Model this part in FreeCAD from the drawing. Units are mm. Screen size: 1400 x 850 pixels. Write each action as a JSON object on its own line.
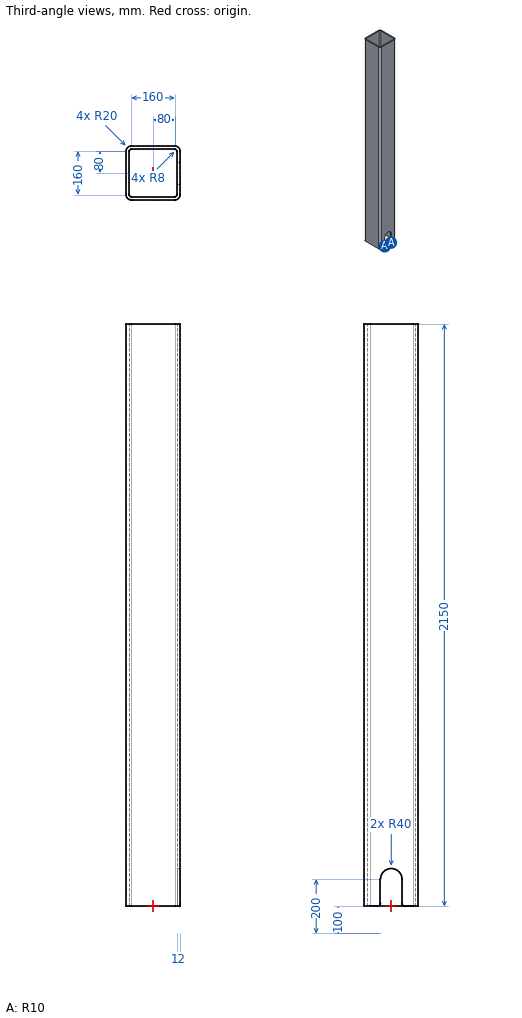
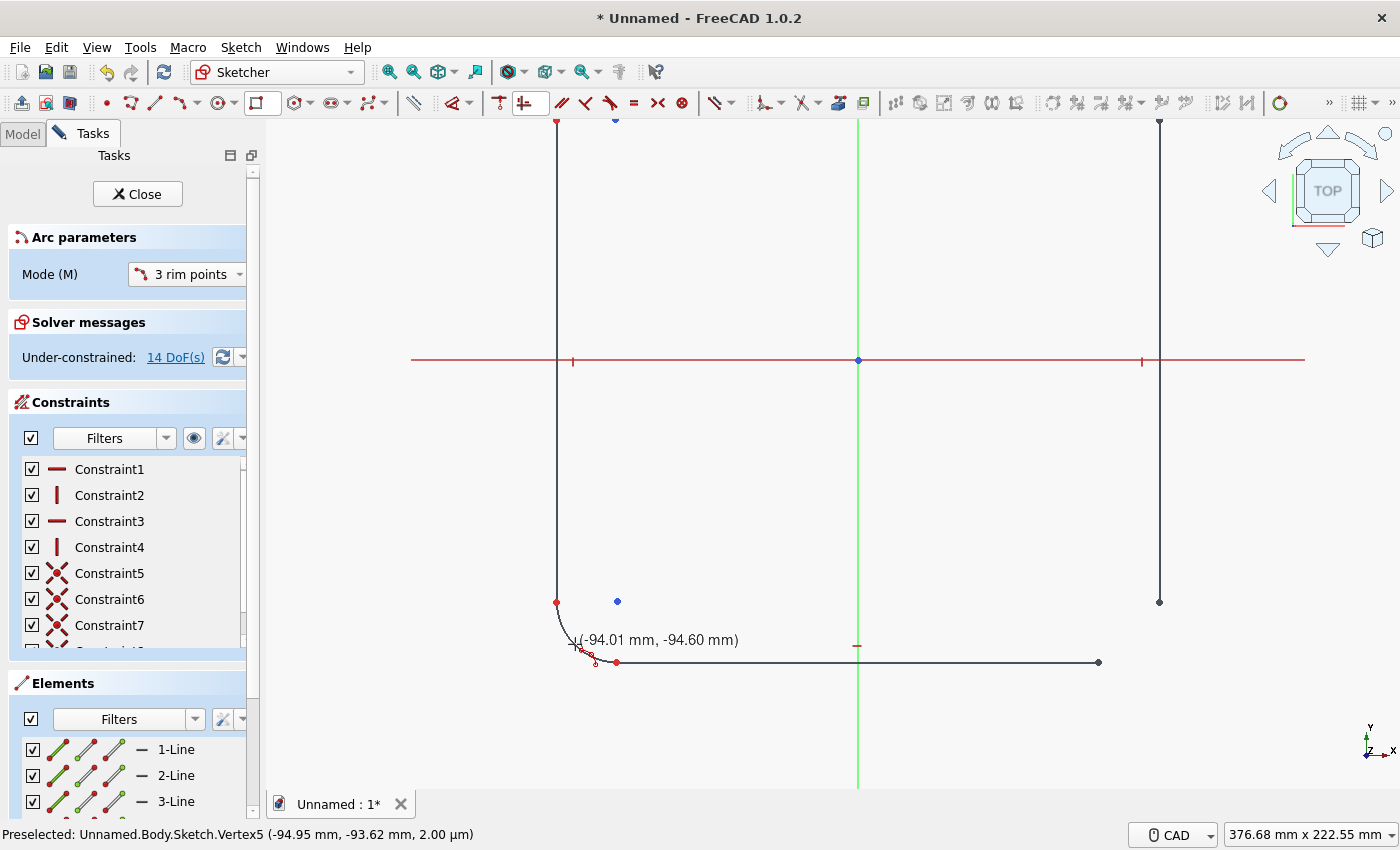
{"action": "left_click", "coordinate": [1098, 663]}
{"action": "left_click", "coordinate": [1160, 603]}
{"action": "left_click", "coordinate": [1141, 644]}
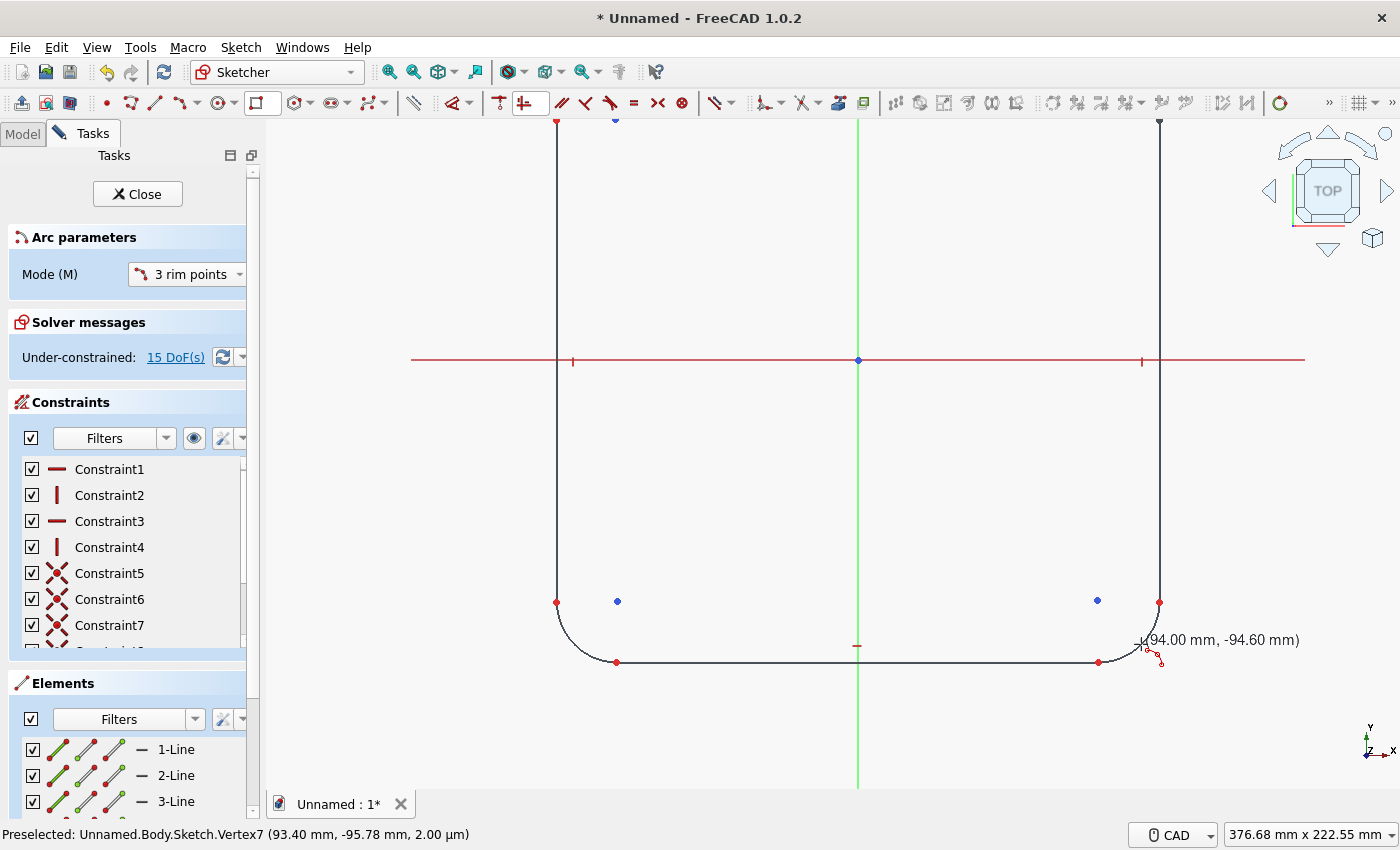
{"action": "scroll", "coordinate": [574, 645], "scroll_direction": "down", "scroll_amount": 2}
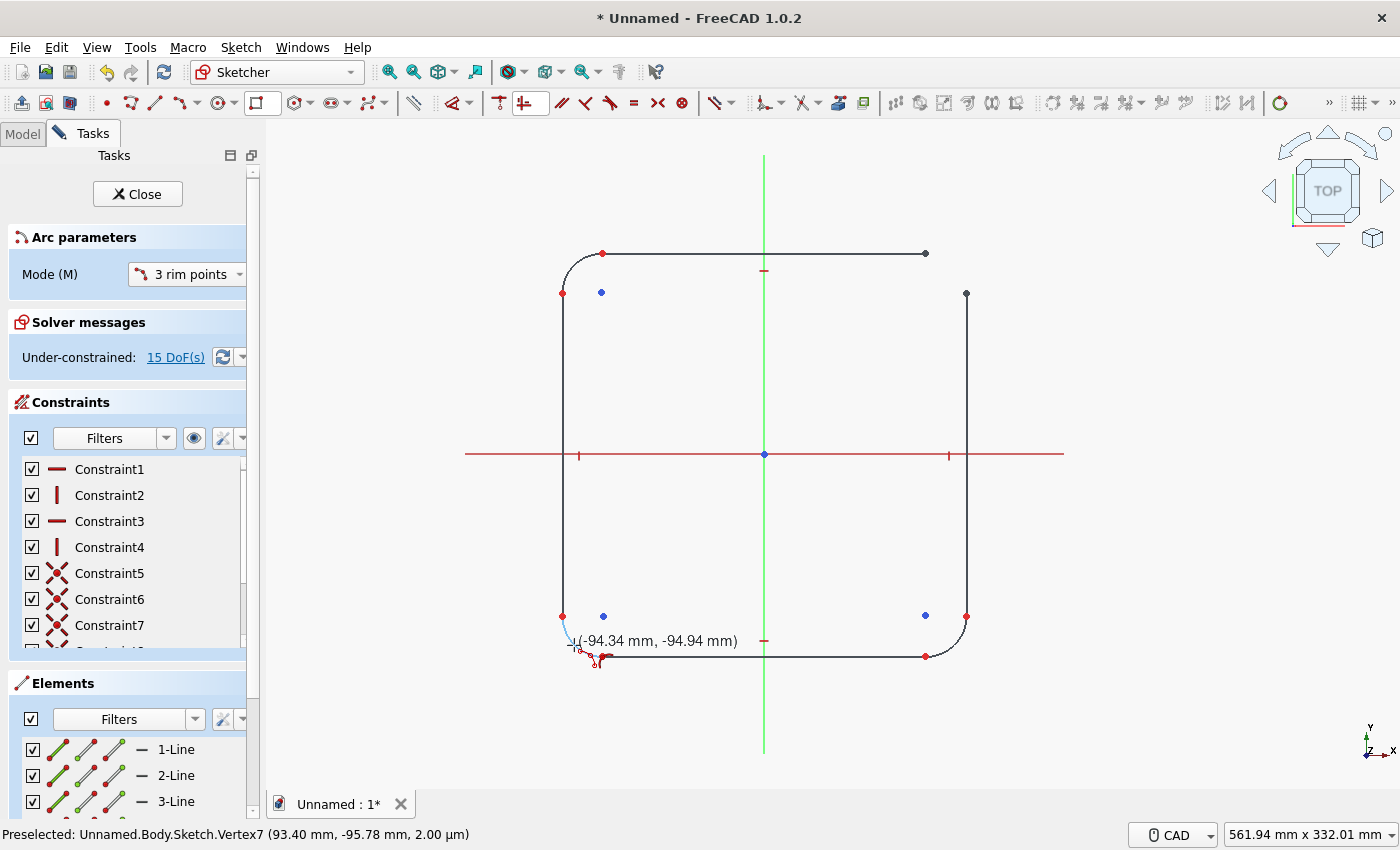
{"action": "left_click", "coordinate": [967, 294]}
{"action": "left_click", "coordinate": [926, 254]}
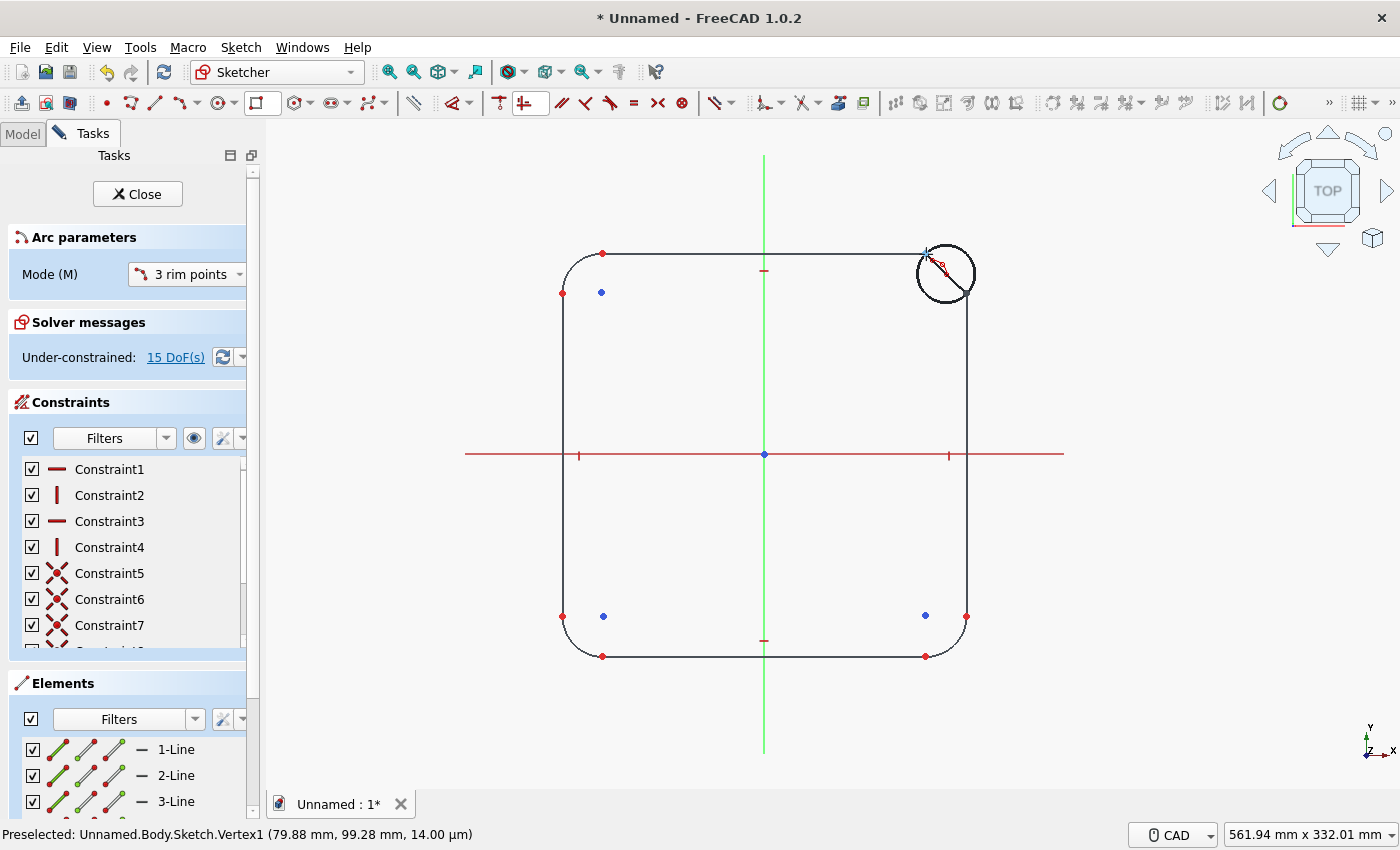
{"action": "scroll", "coordinate": [954, 264], "scroll_direction": "up", "scroll_amount": 2}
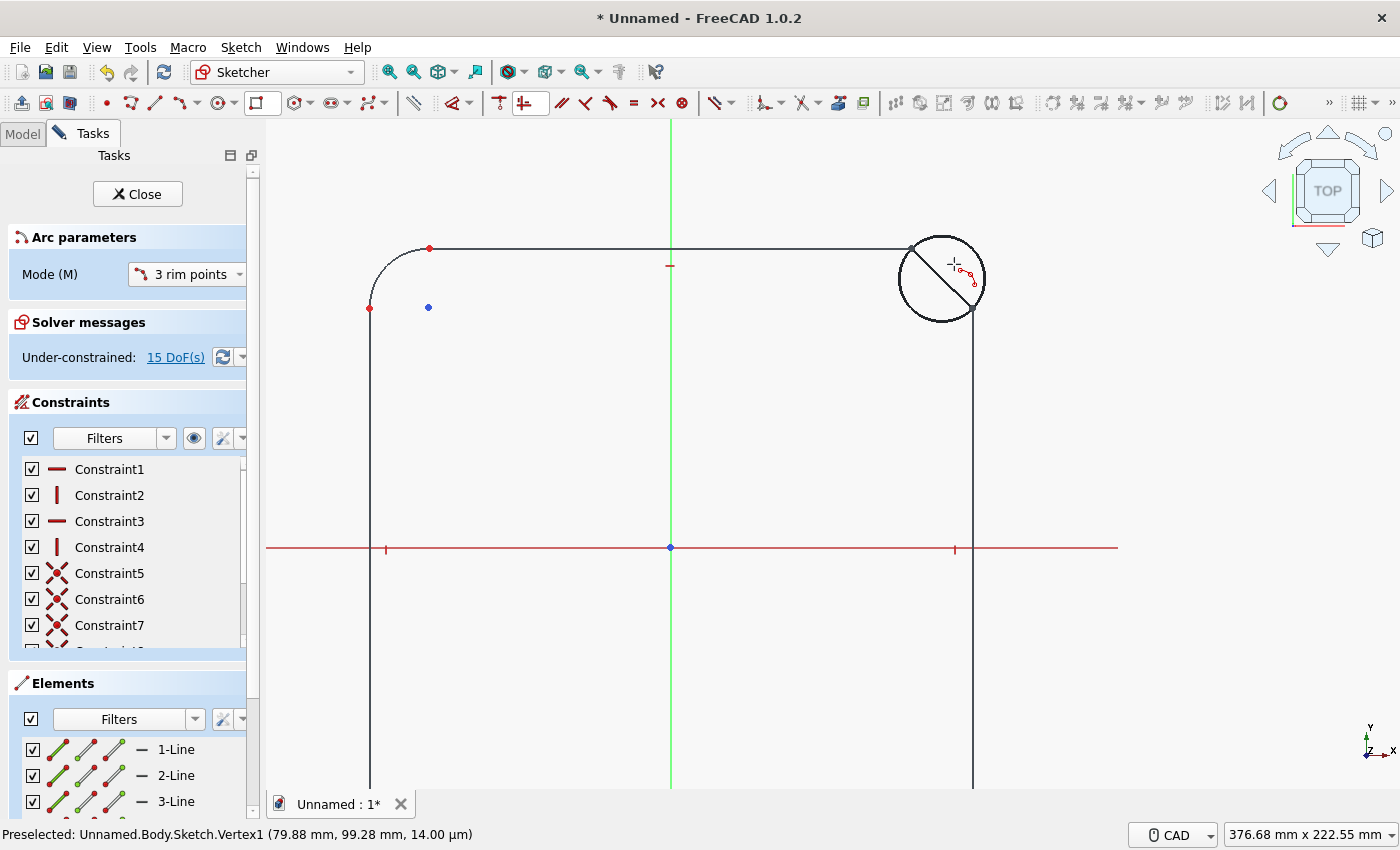
{"action": "left_click", "coordinate": [954, 264]}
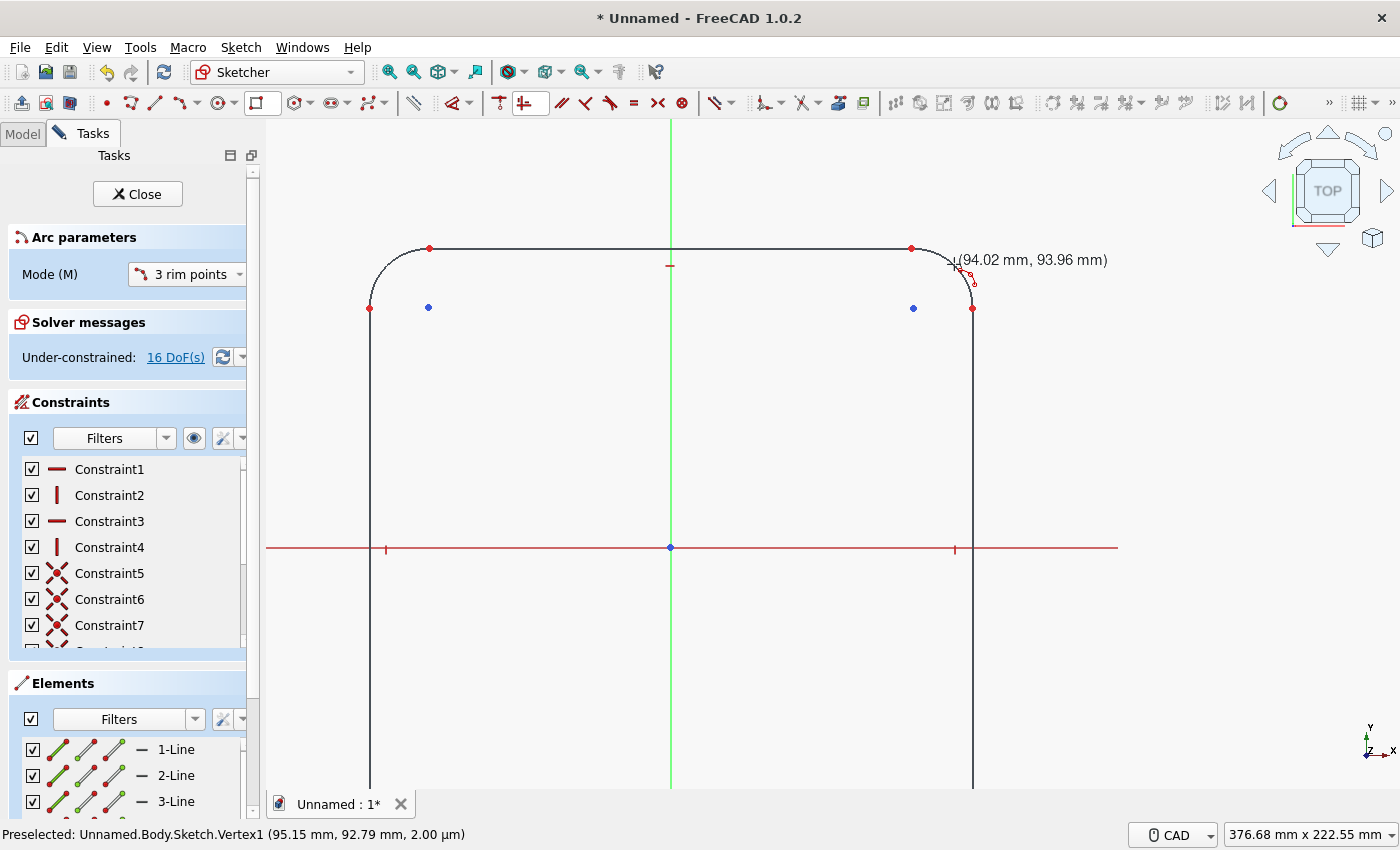
{"action": "left_click", "coordinate": [156, 104]}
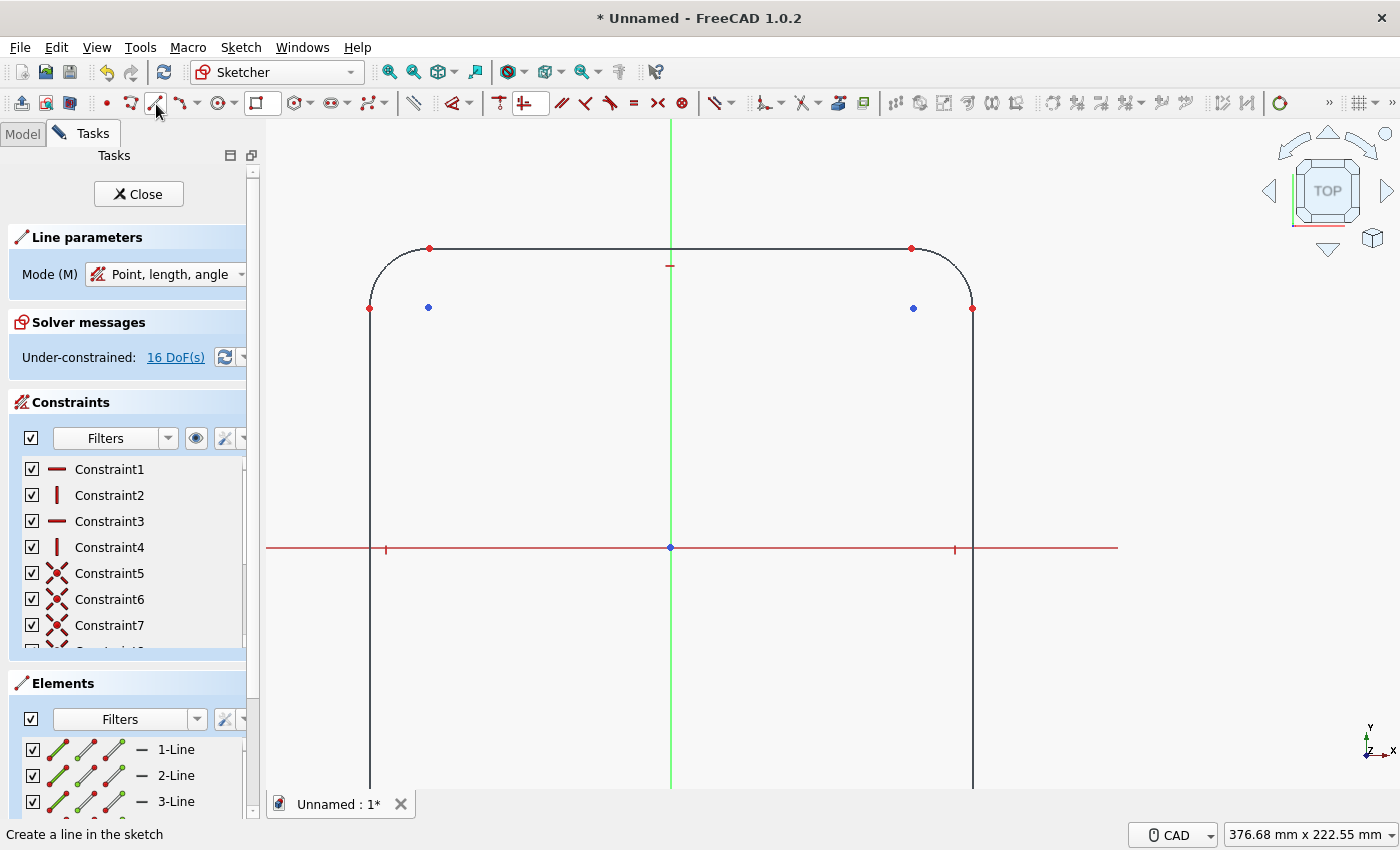
{"action": "left_click", "coordinate": [430, 283]}
{"action": "left_click", "coordinate": [912, 283]}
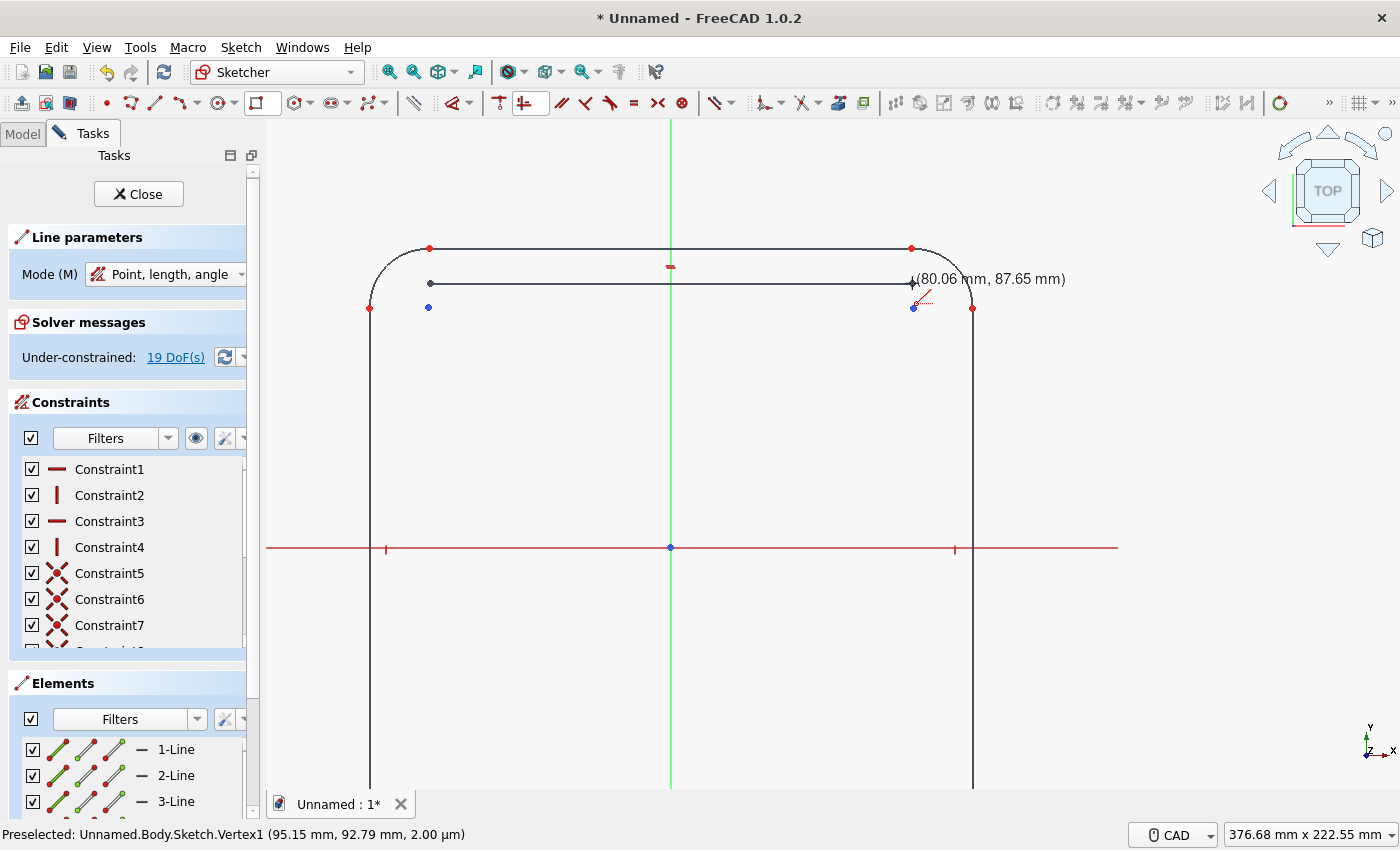
{"action": "left_click", "coordinate": [936, 307]}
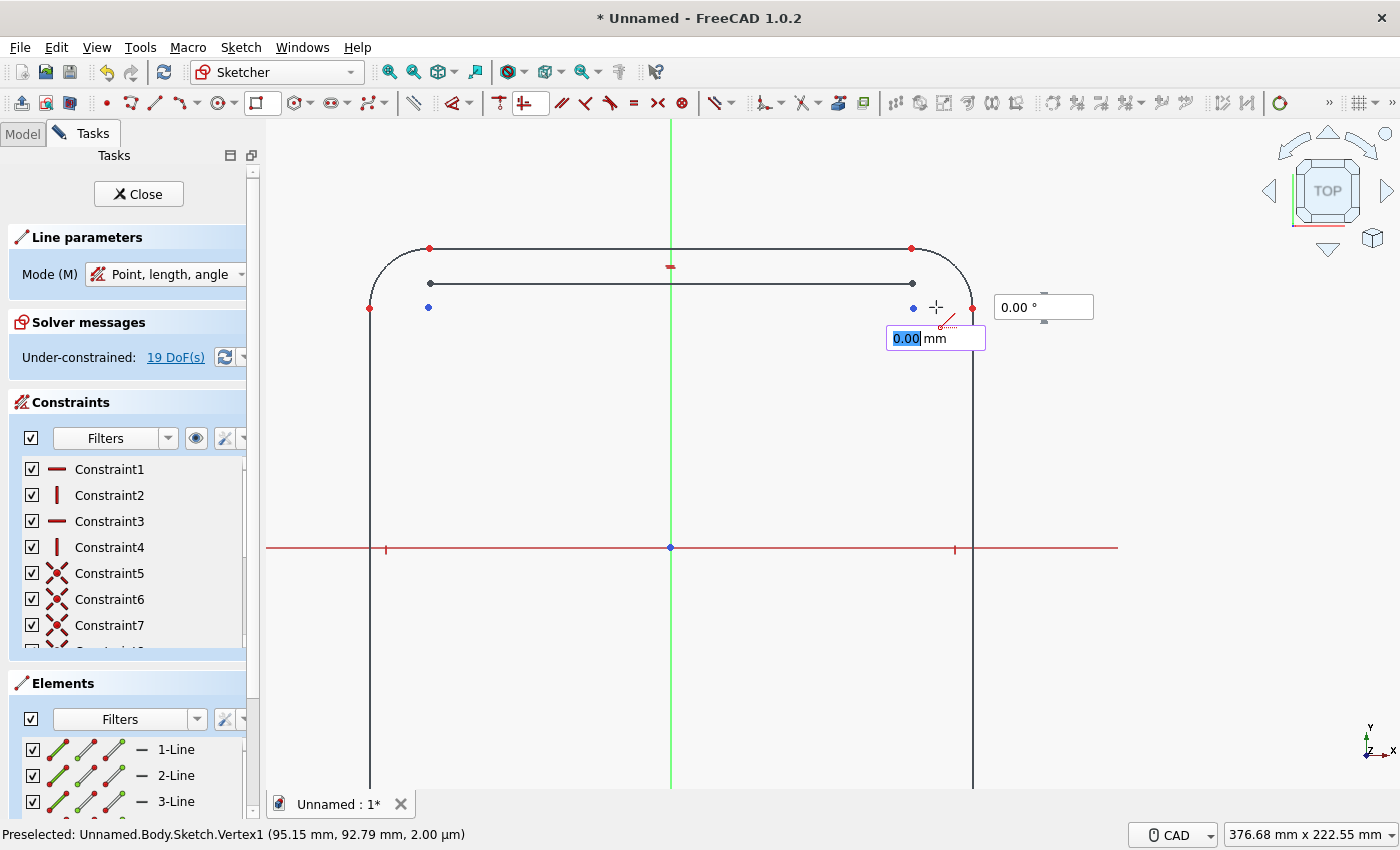
{"action": "scroll", "coordinate": [955, 263], "scroll_direction": "down", "scroll_amount": 2}